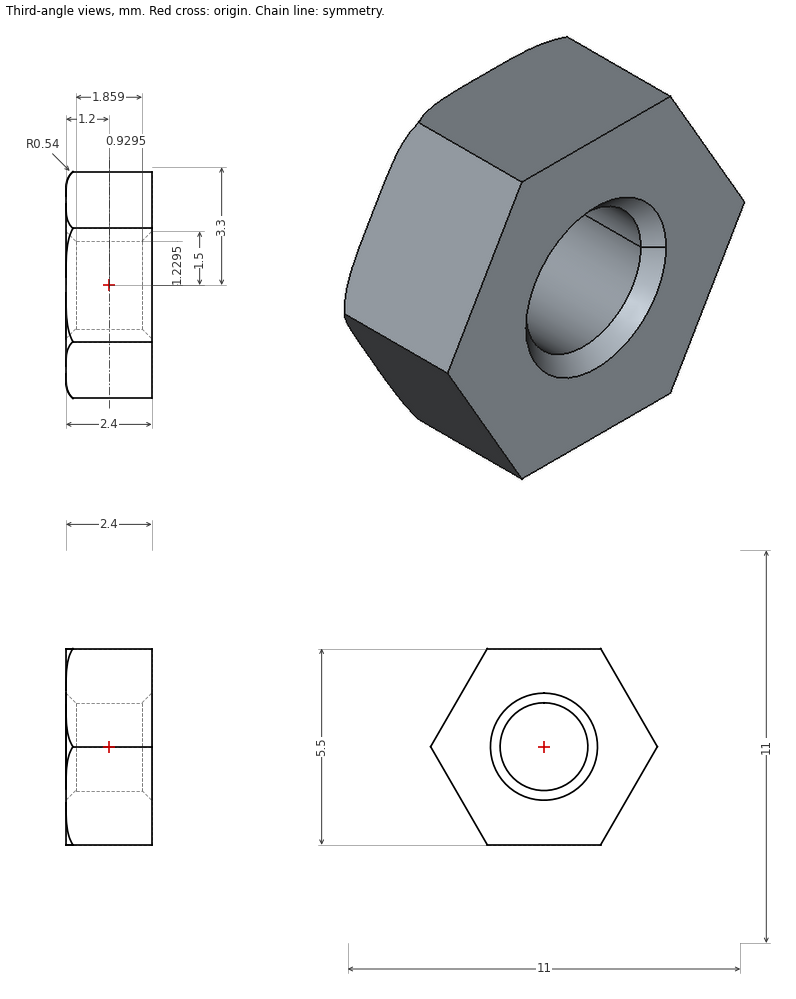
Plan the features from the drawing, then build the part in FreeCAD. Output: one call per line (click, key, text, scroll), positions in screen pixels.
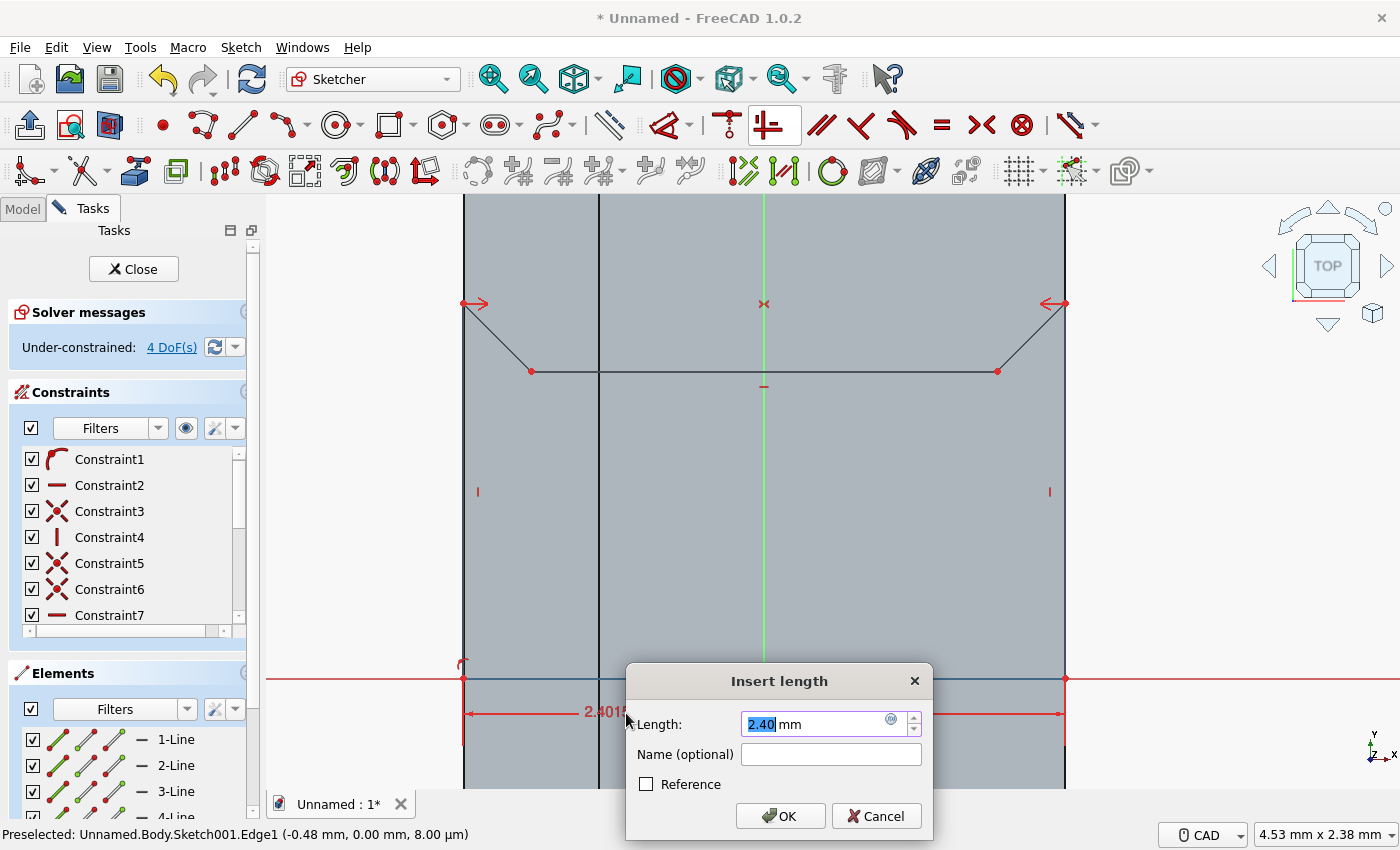
text(2.4)
key(Return)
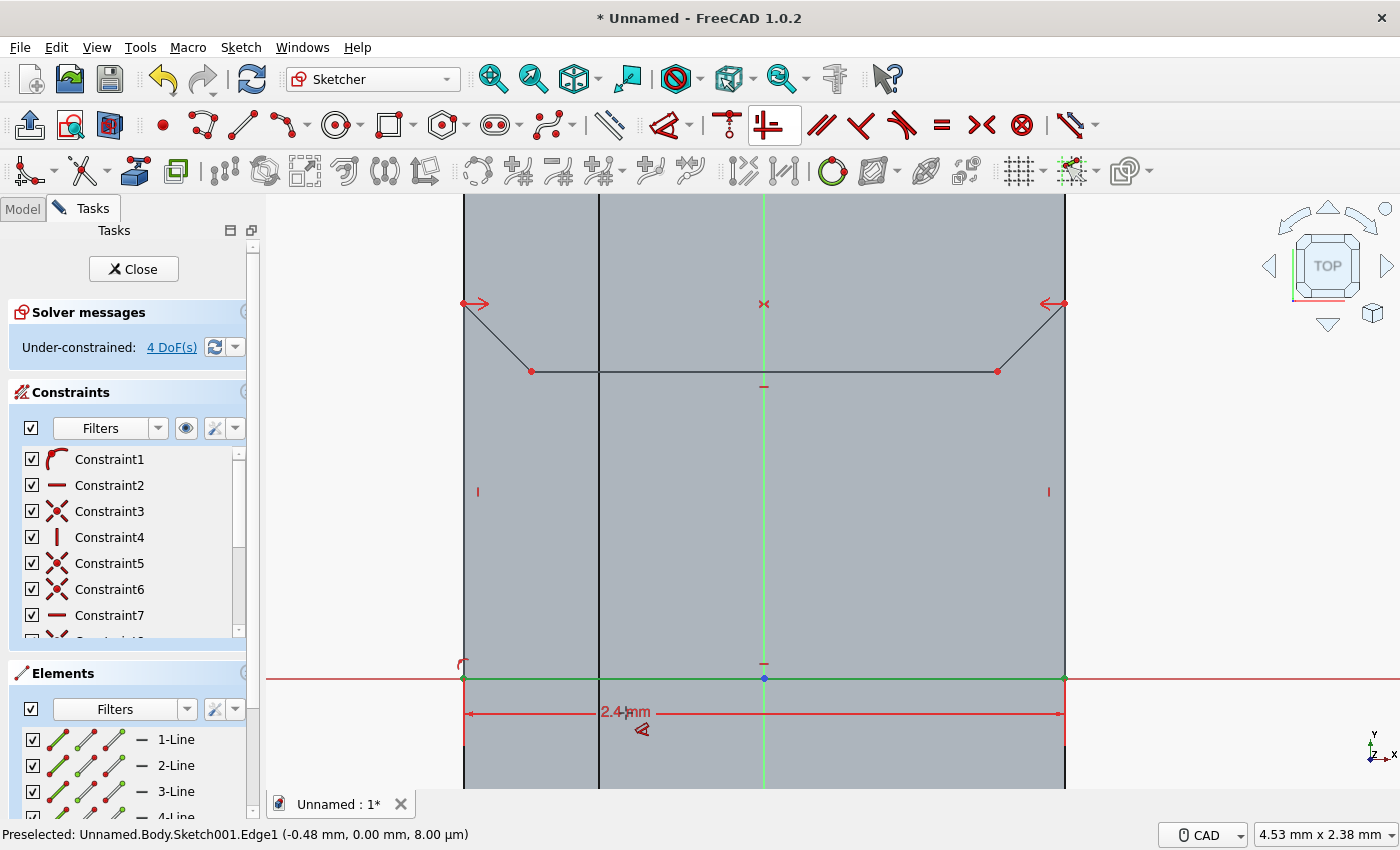
click(1065, 566)
click(1099, 491)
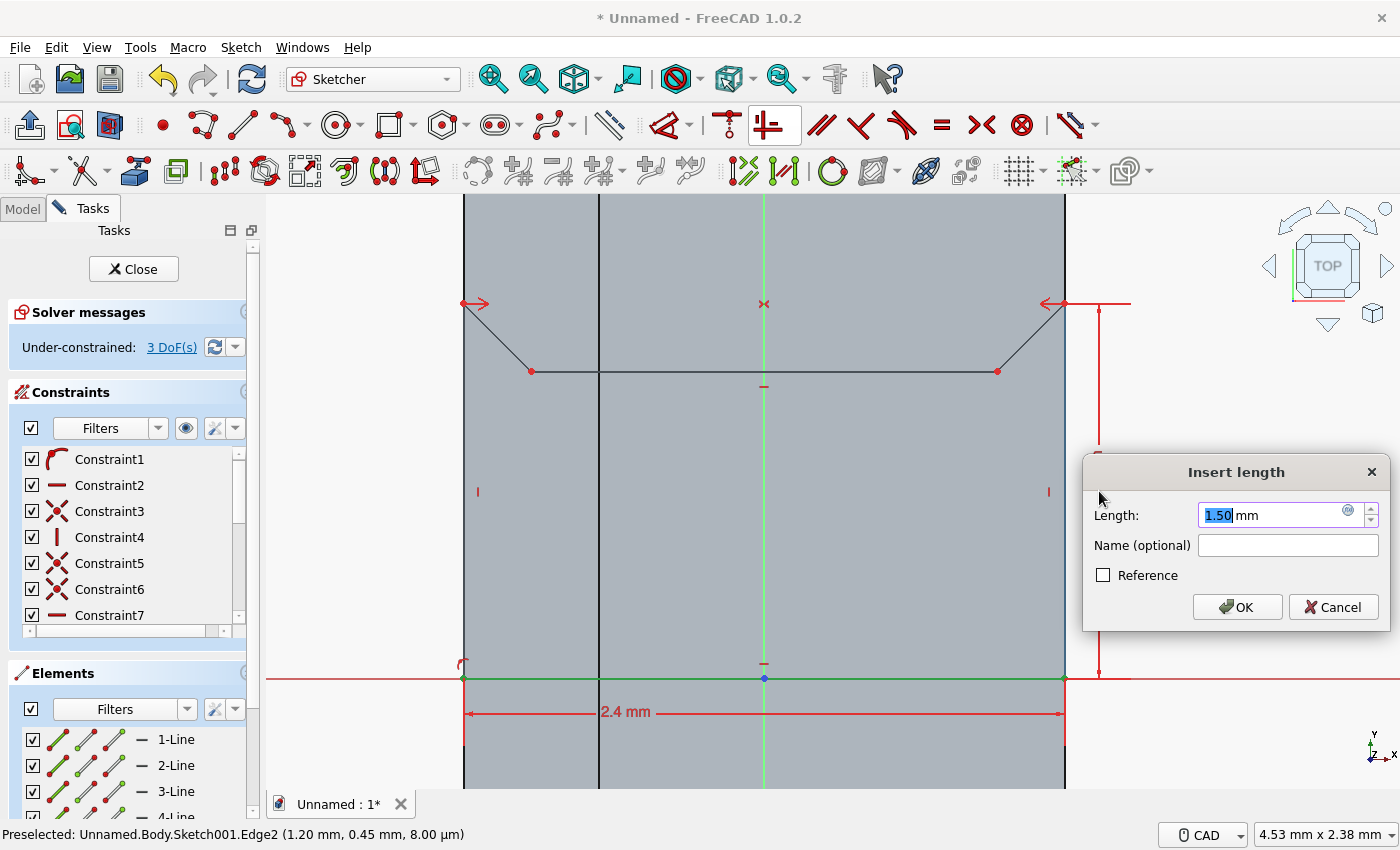
text(1.5)
key(Return)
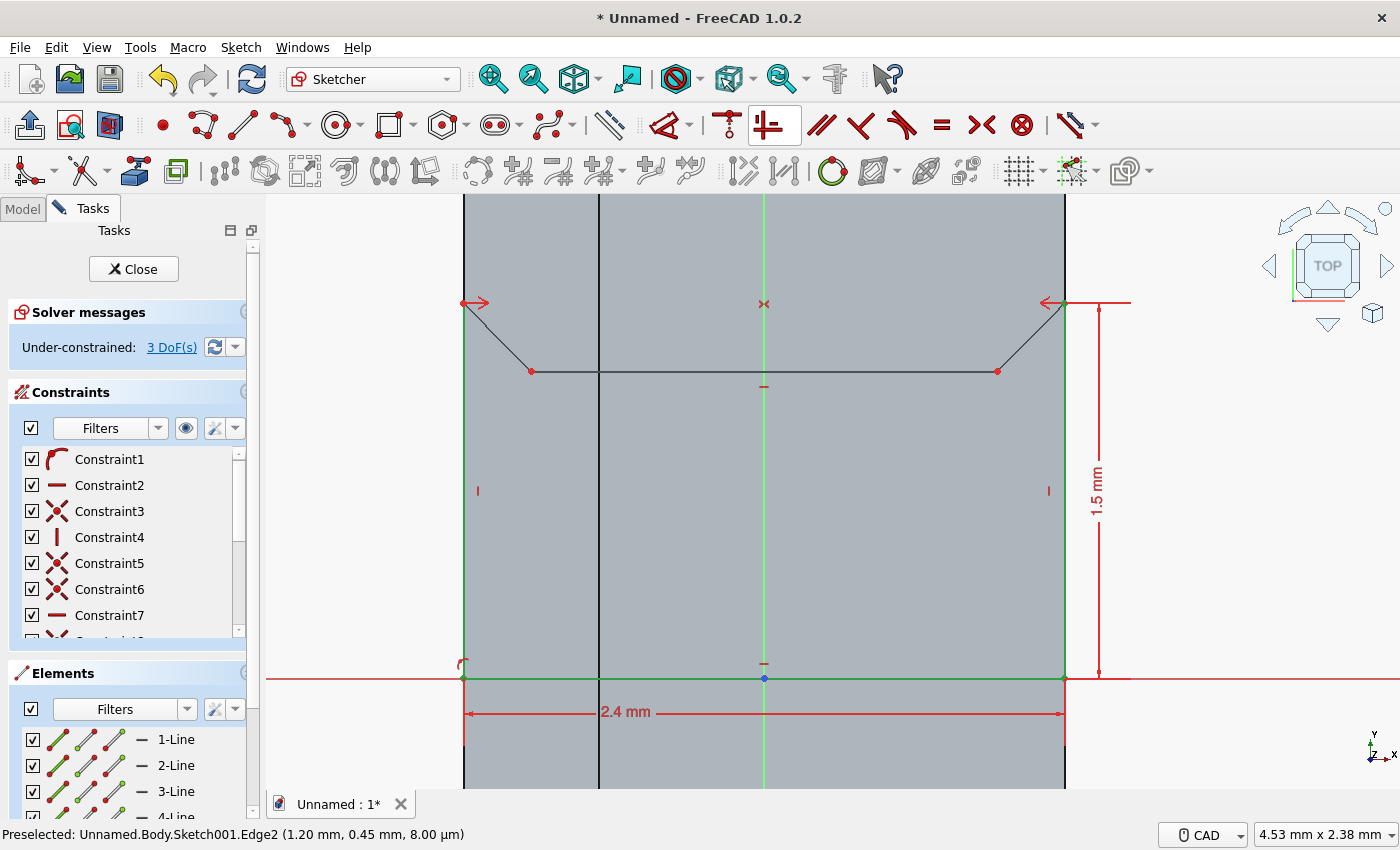
click(857, 372)
click(657, 338)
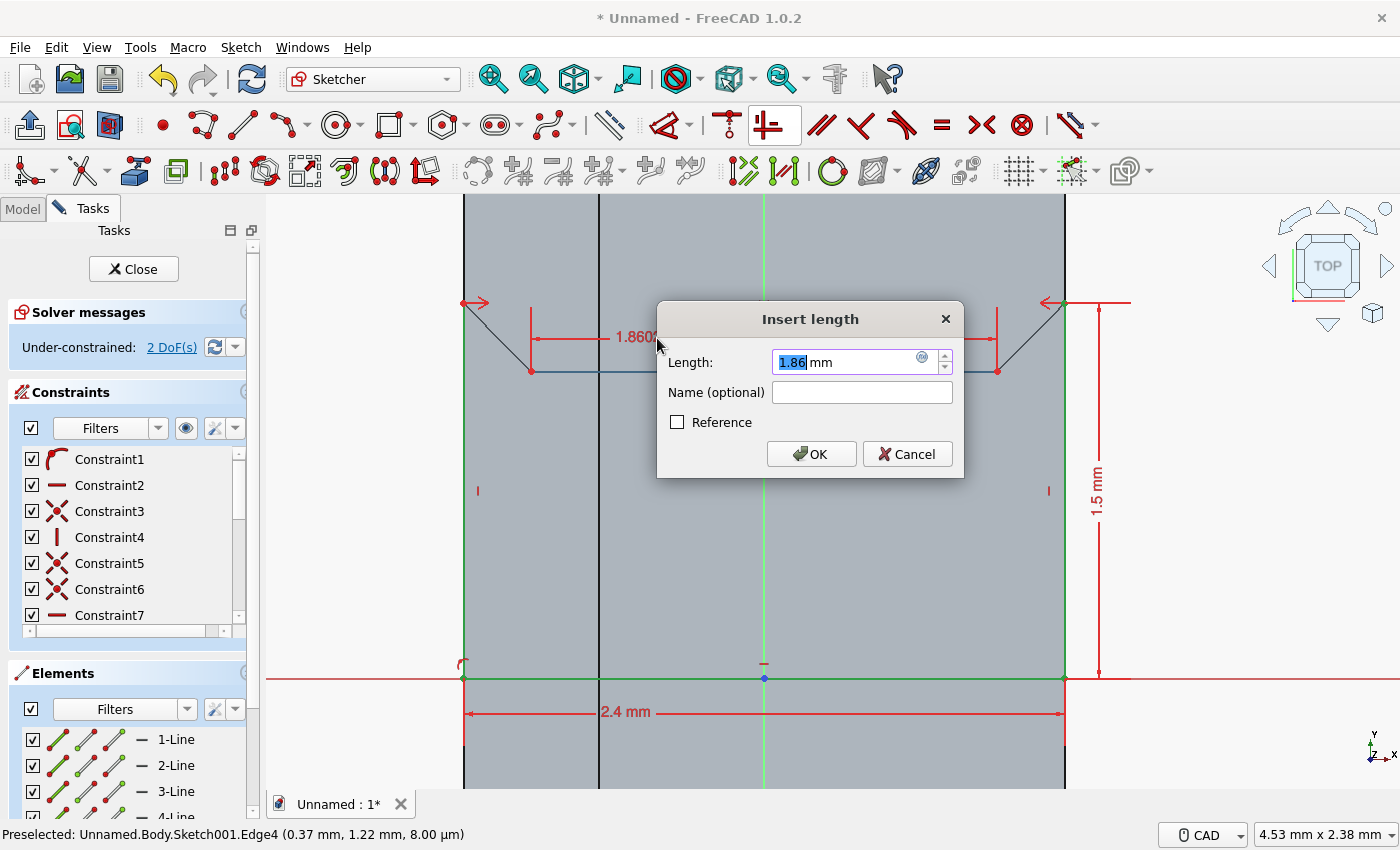
text(1.859)
key(Return)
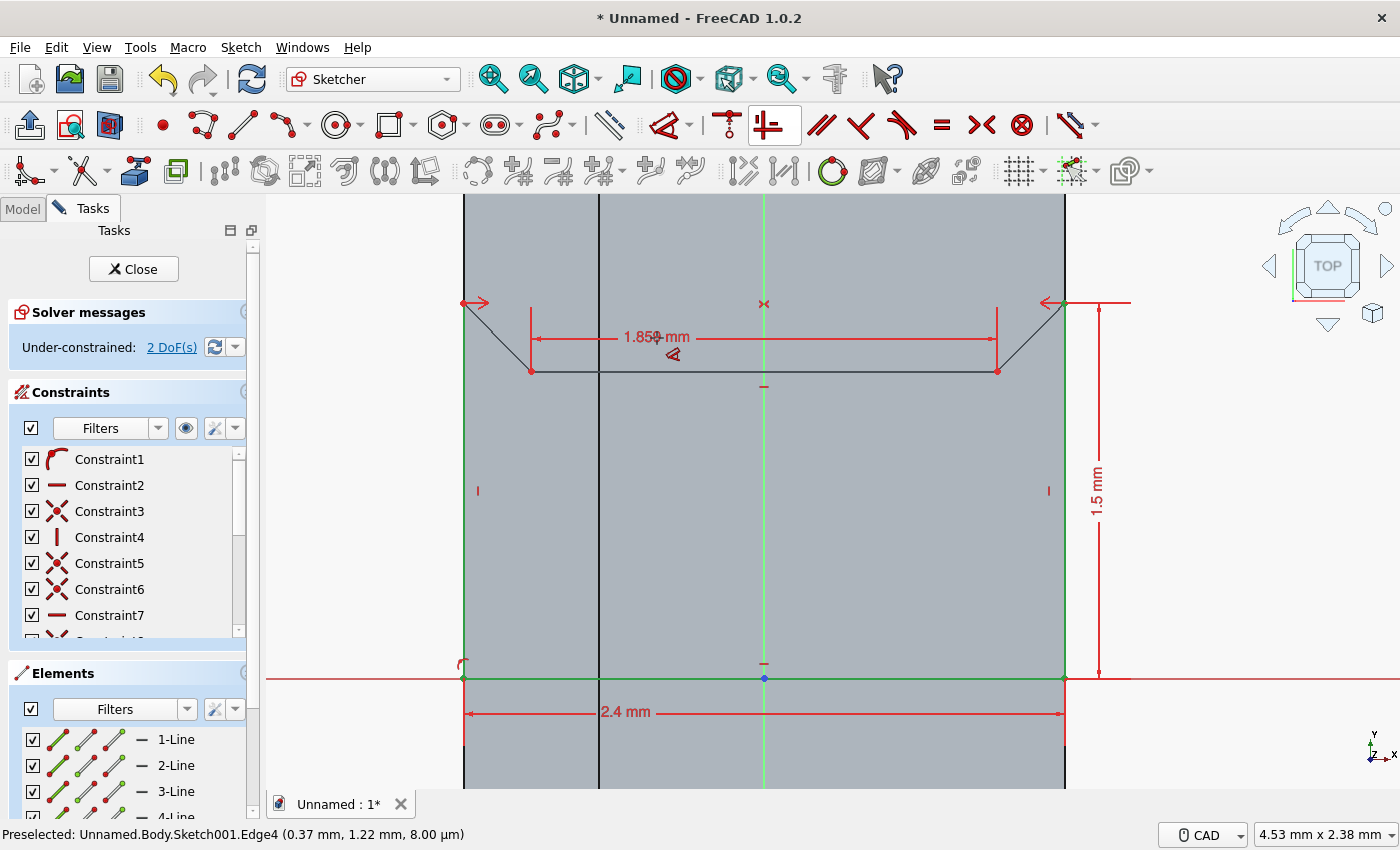
click(997, 372)
click(881, 713)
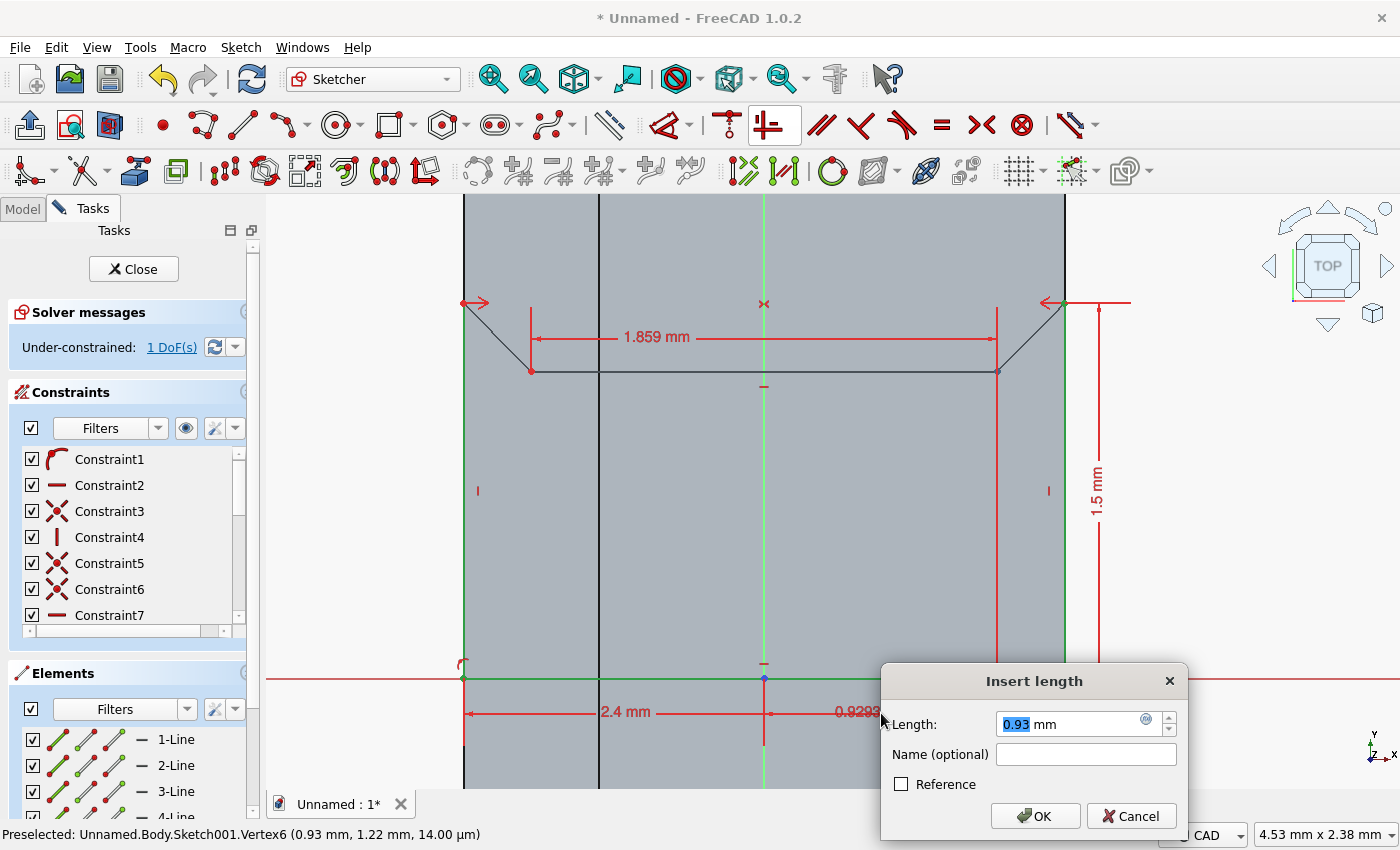
text(0.9295)
key(Return)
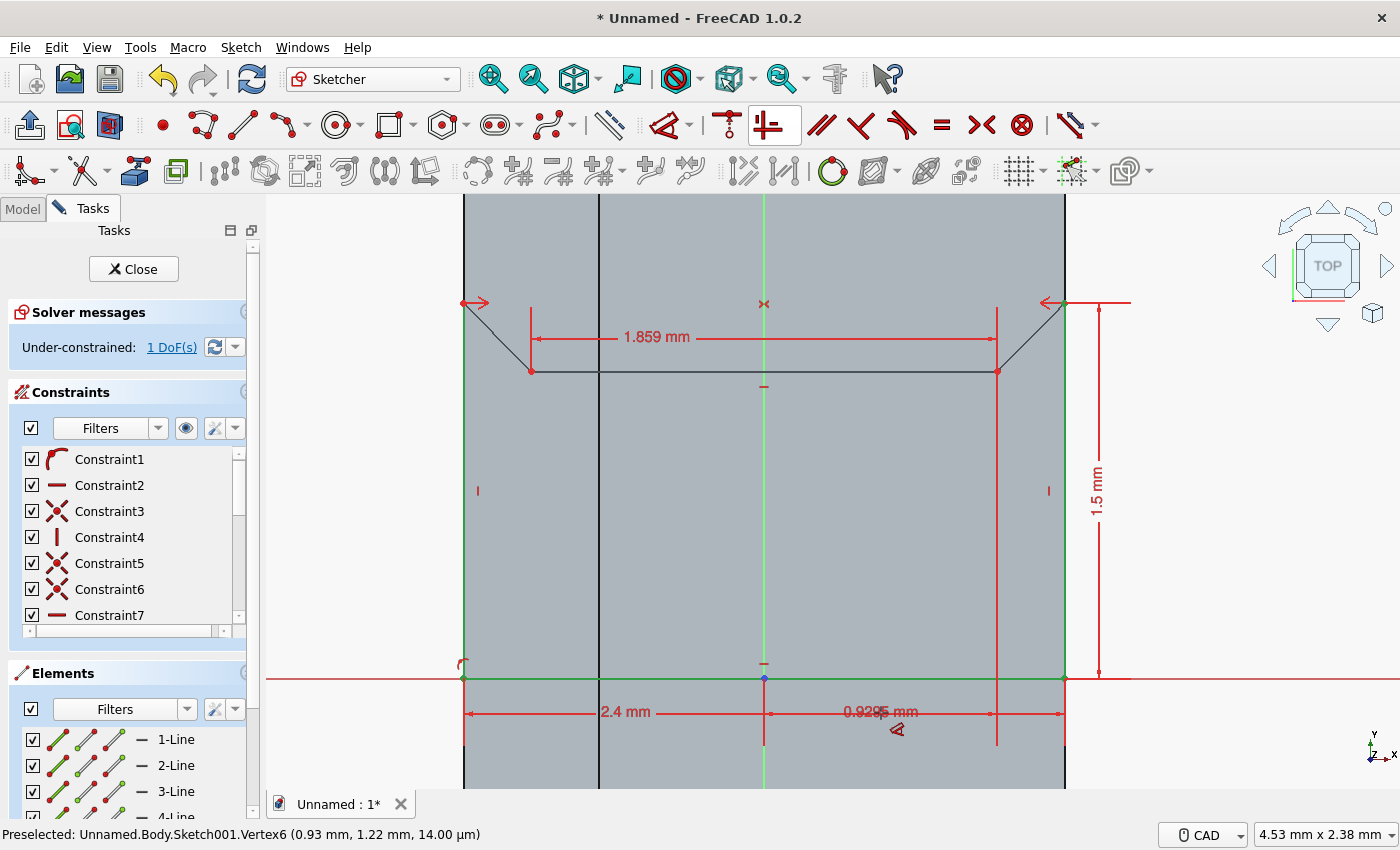
click(997, 372)
click(1031, 525)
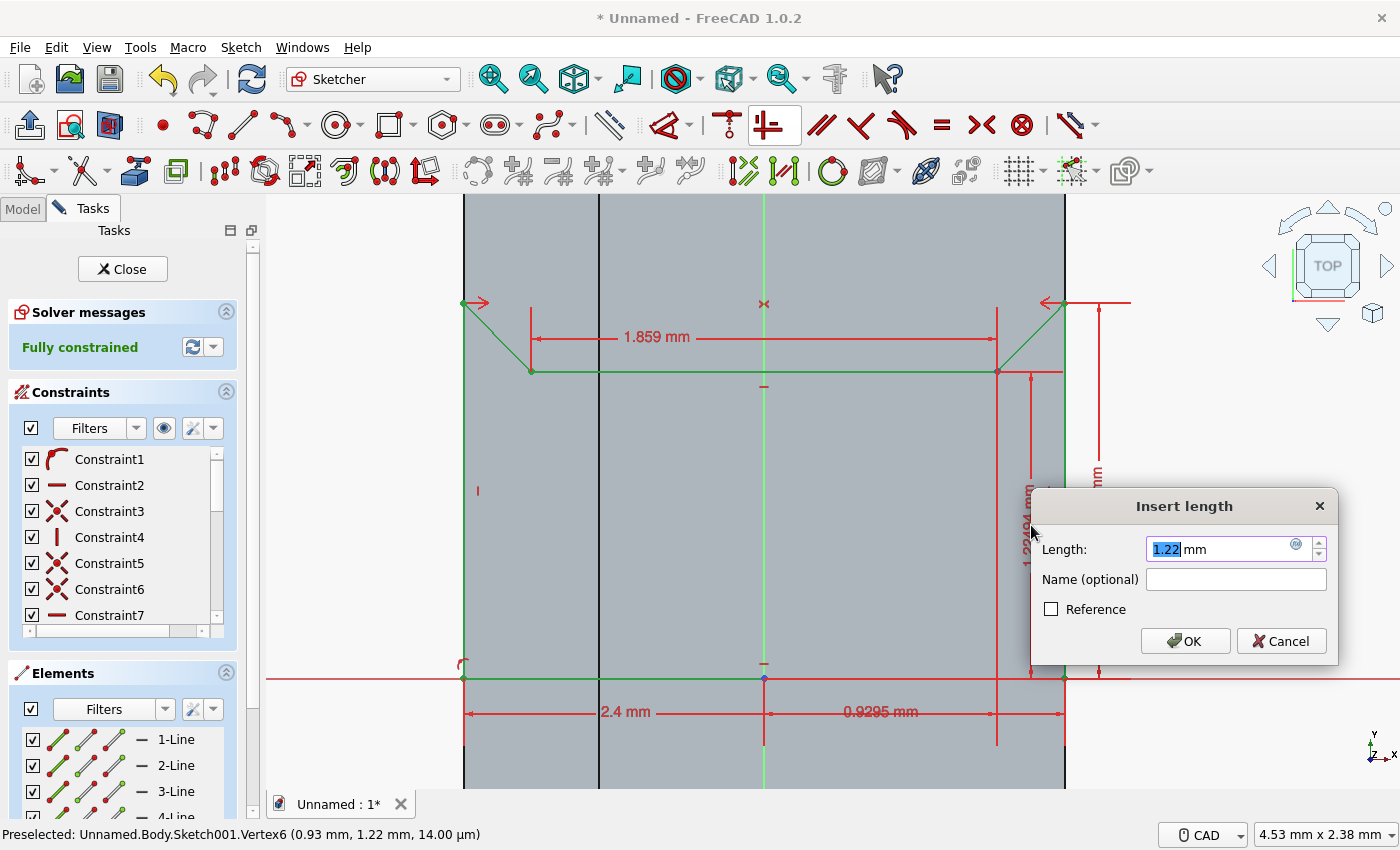
text(1.2295)
key(Return)
key(Escape)